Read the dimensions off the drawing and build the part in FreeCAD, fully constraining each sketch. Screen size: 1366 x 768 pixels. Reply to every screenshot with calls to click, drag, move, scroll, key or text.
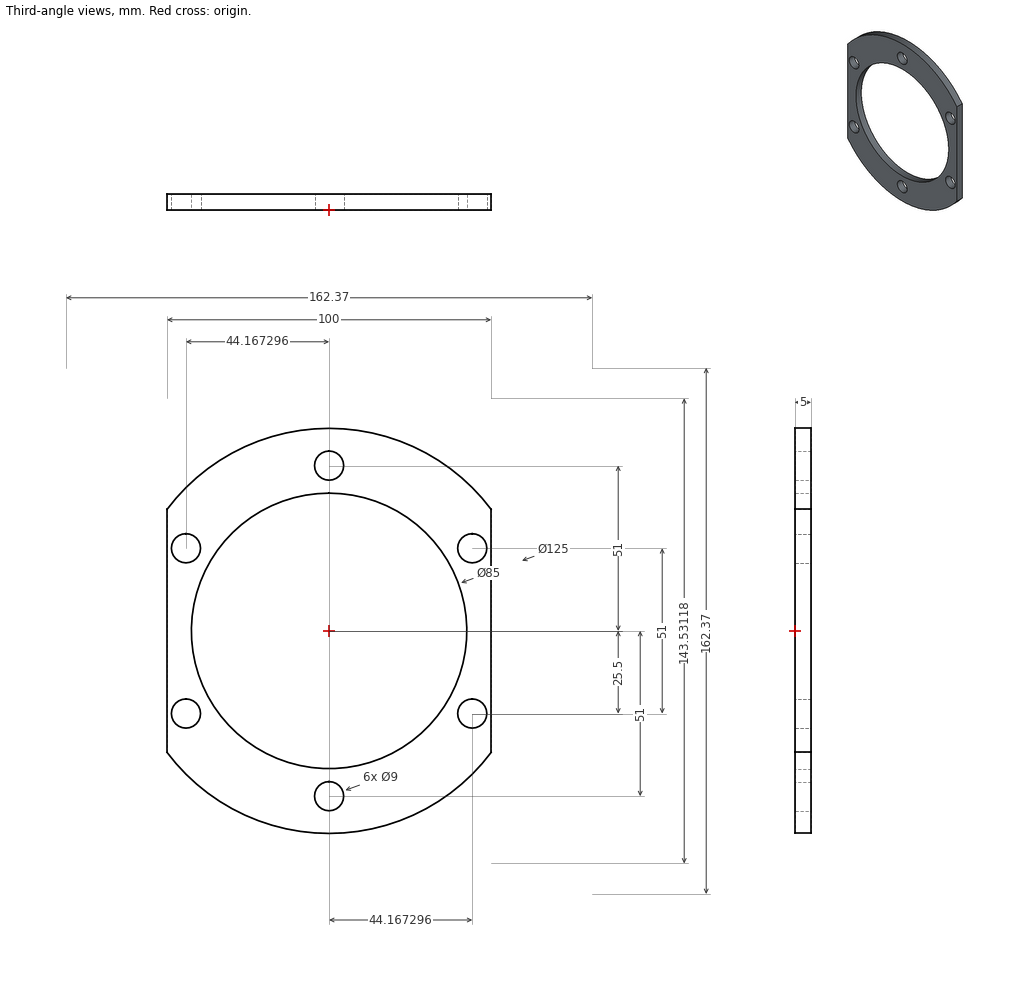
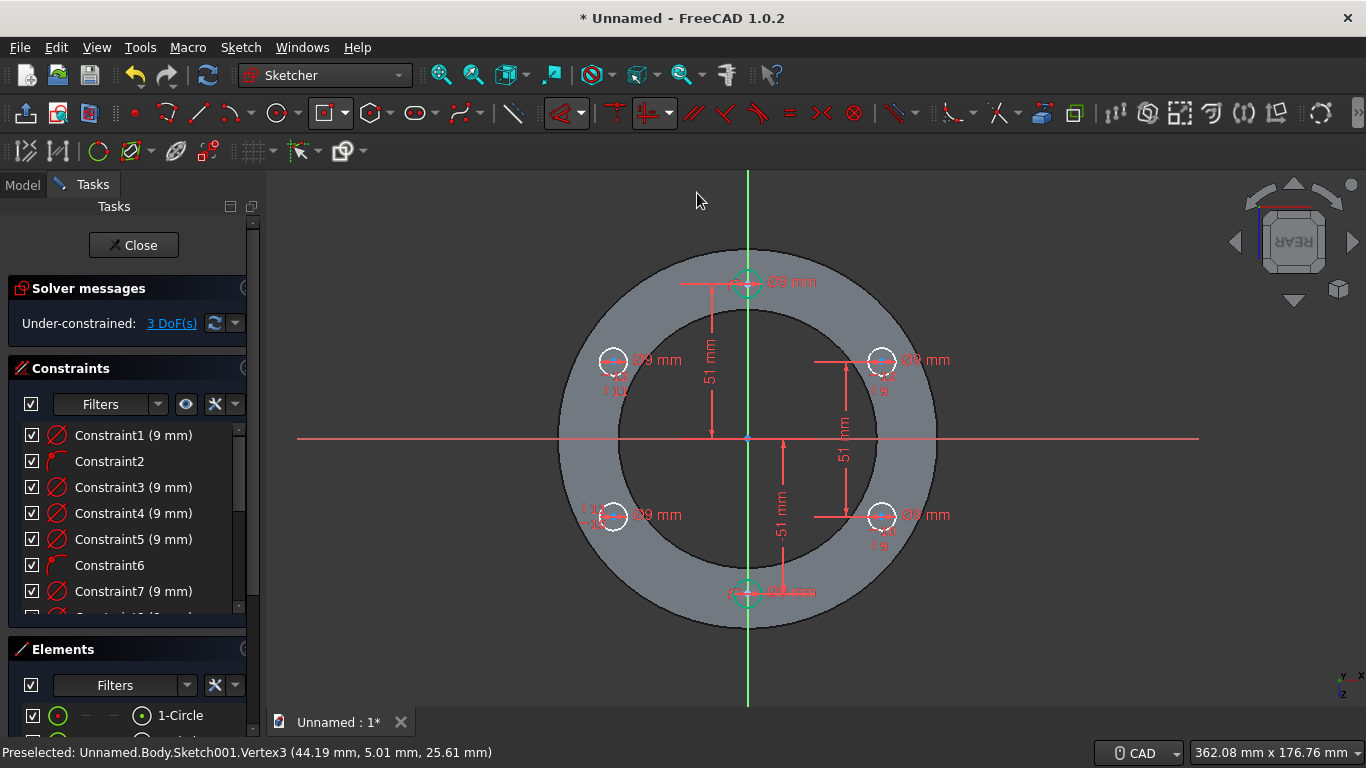
click(882, 362)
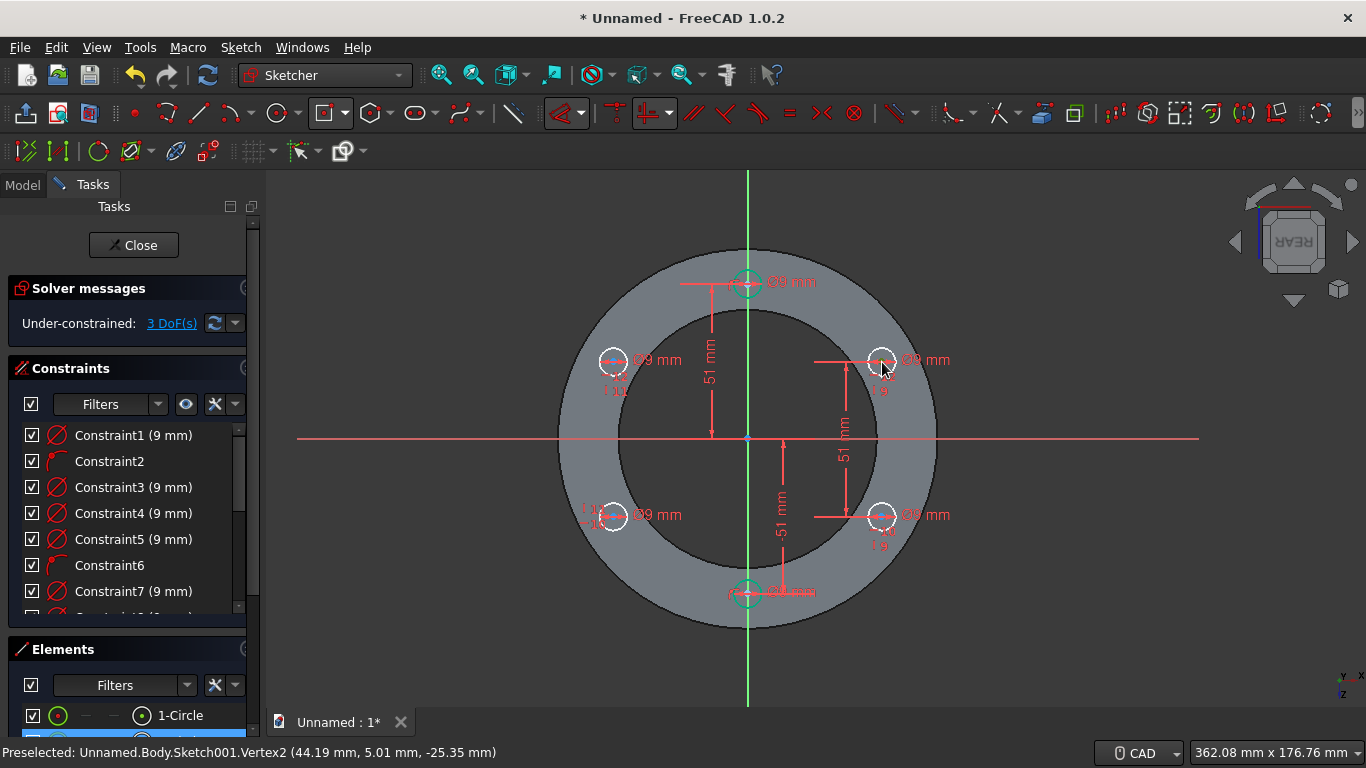
key(i)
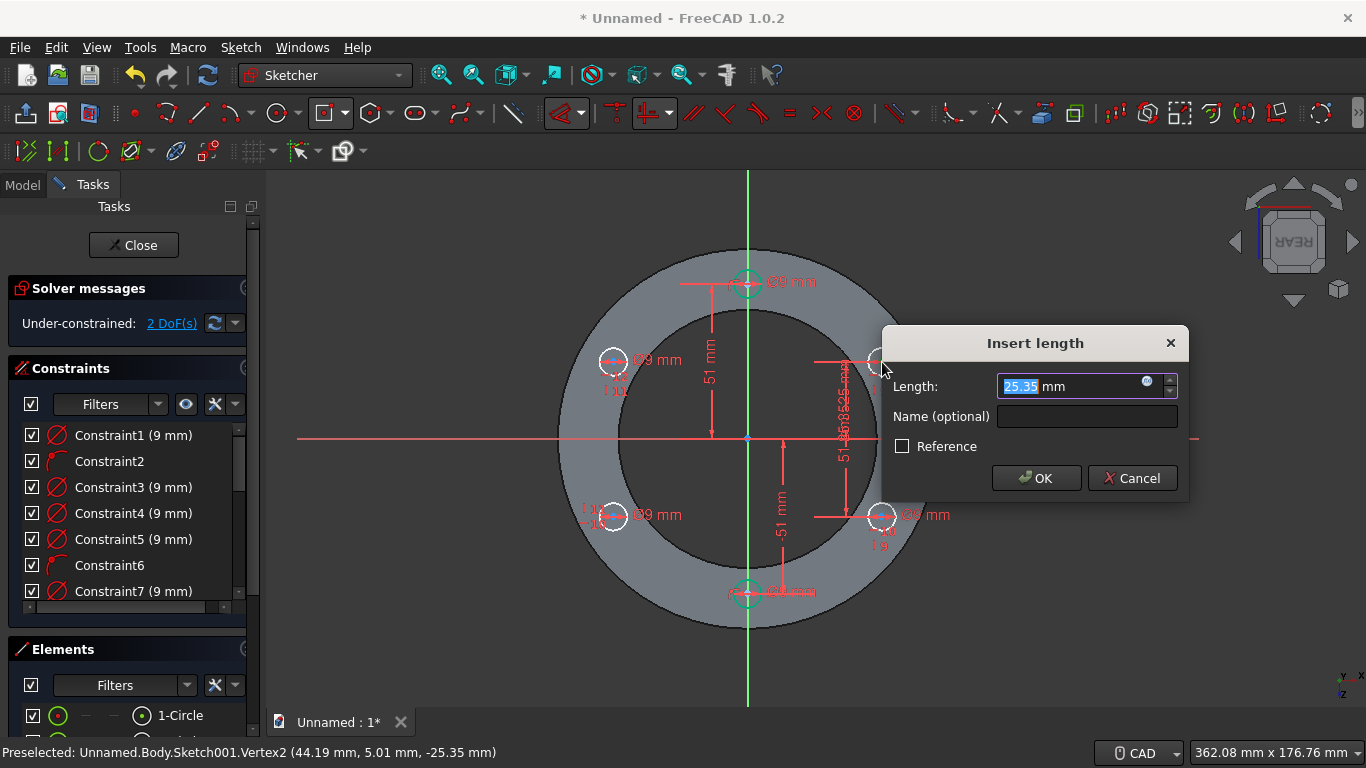
text(25.5)
key(Return)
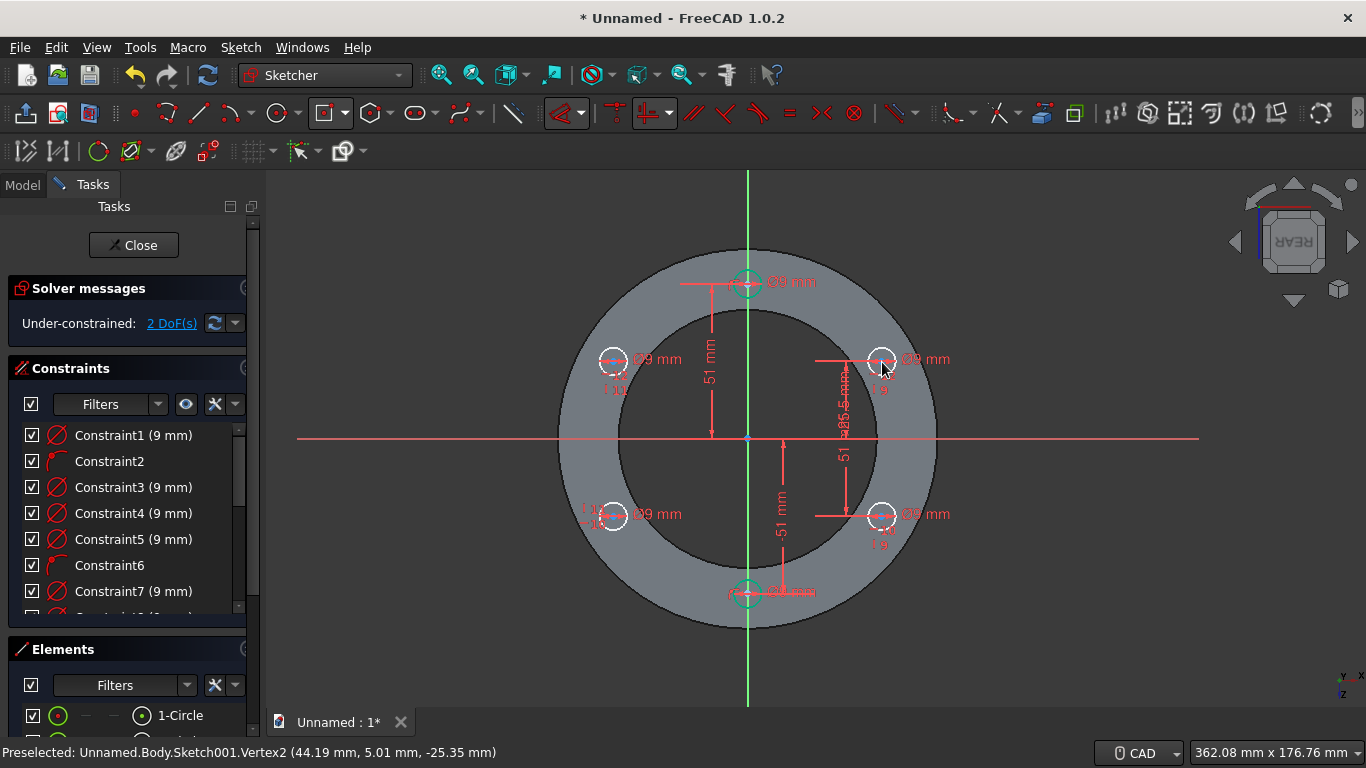
click(882, 361)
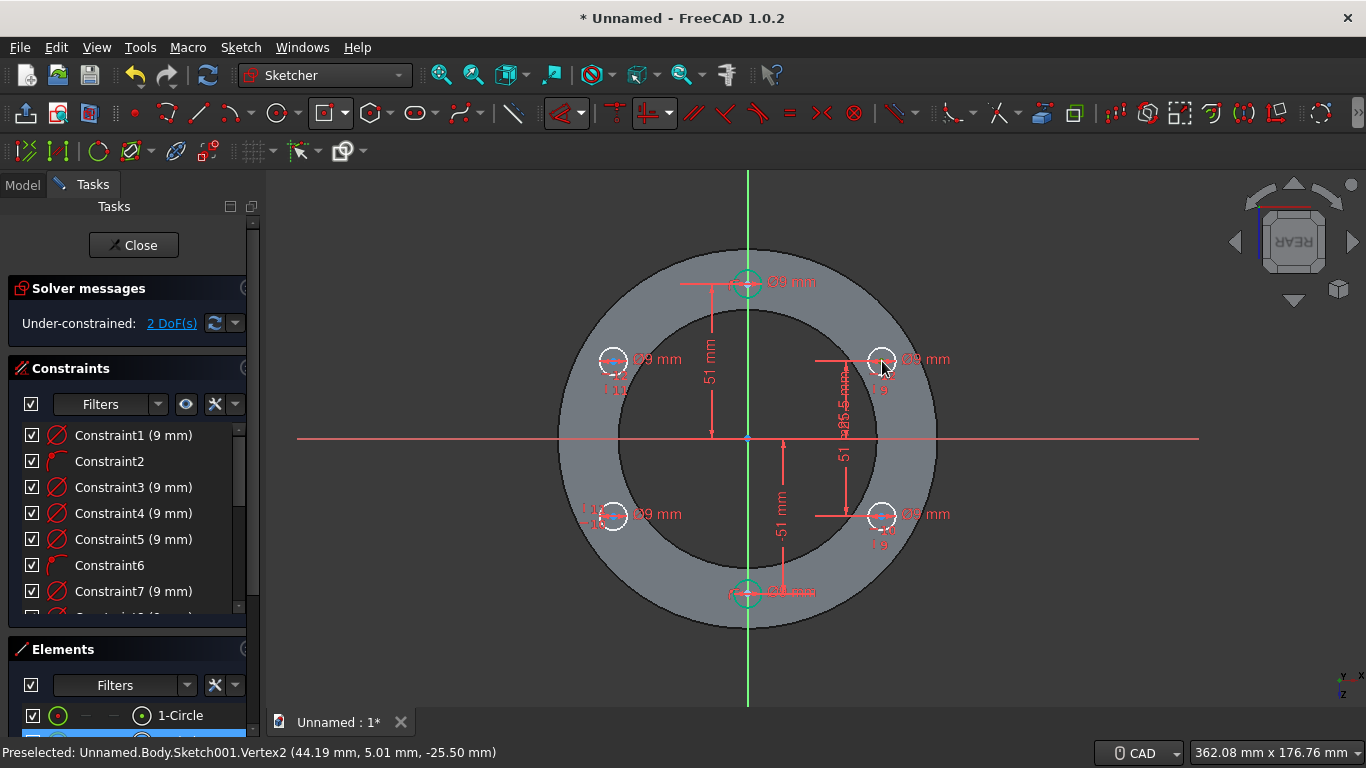
click(584, 114)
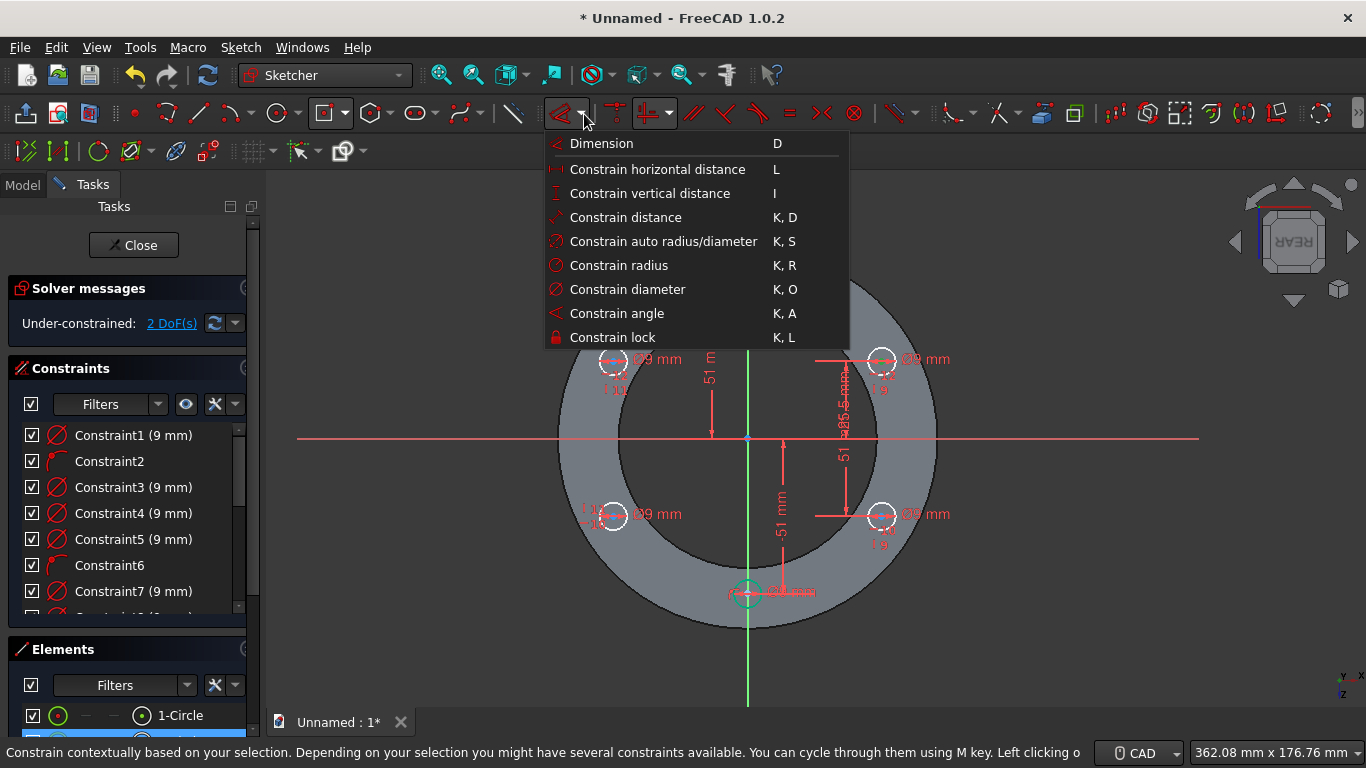
click(697, 169)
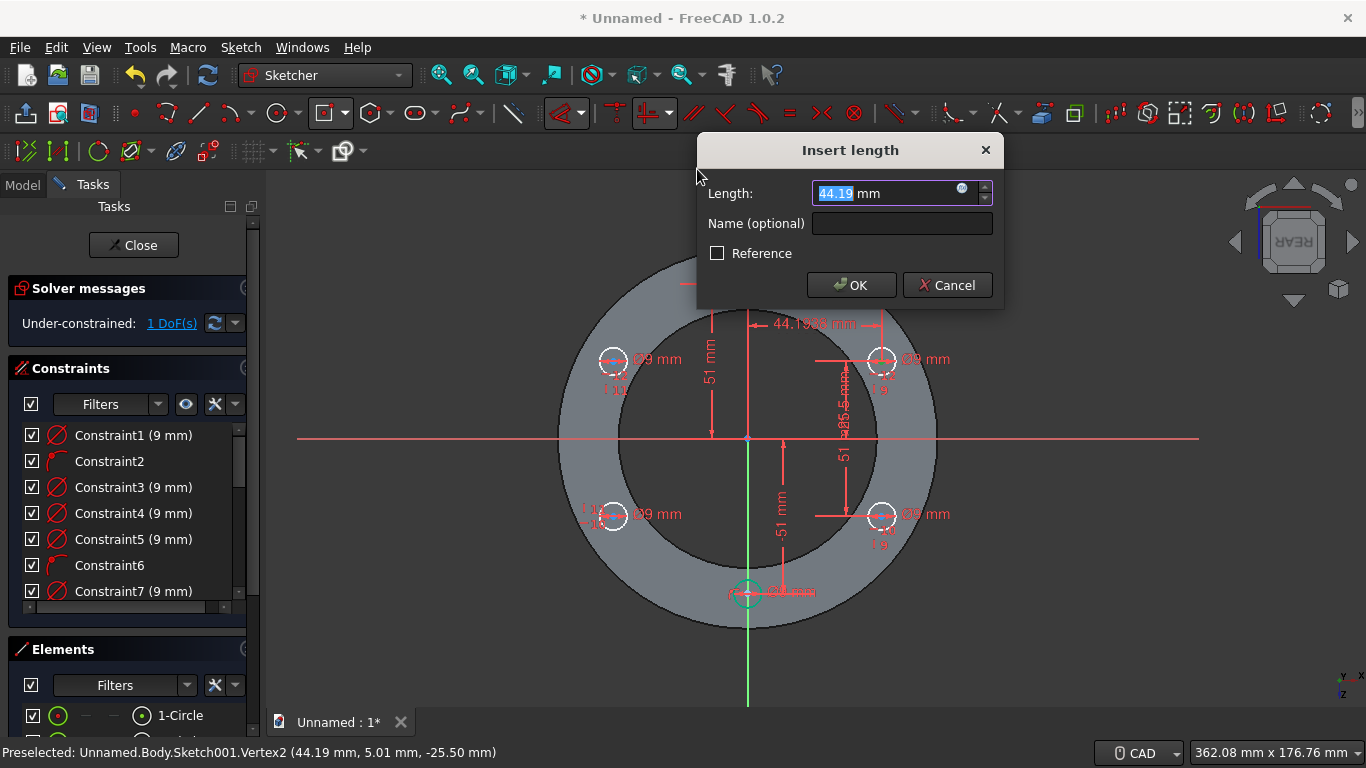
text(44.167296)
key(Return)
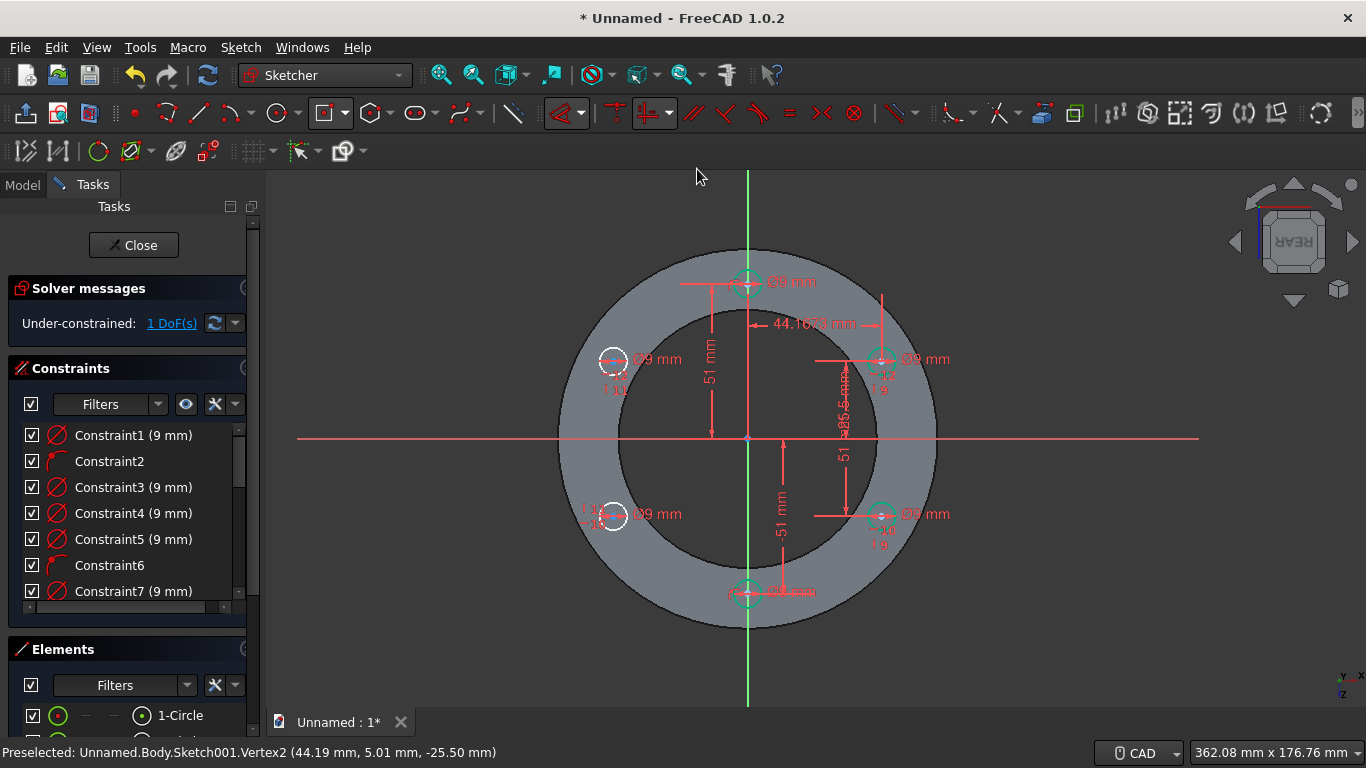
click(613, 516)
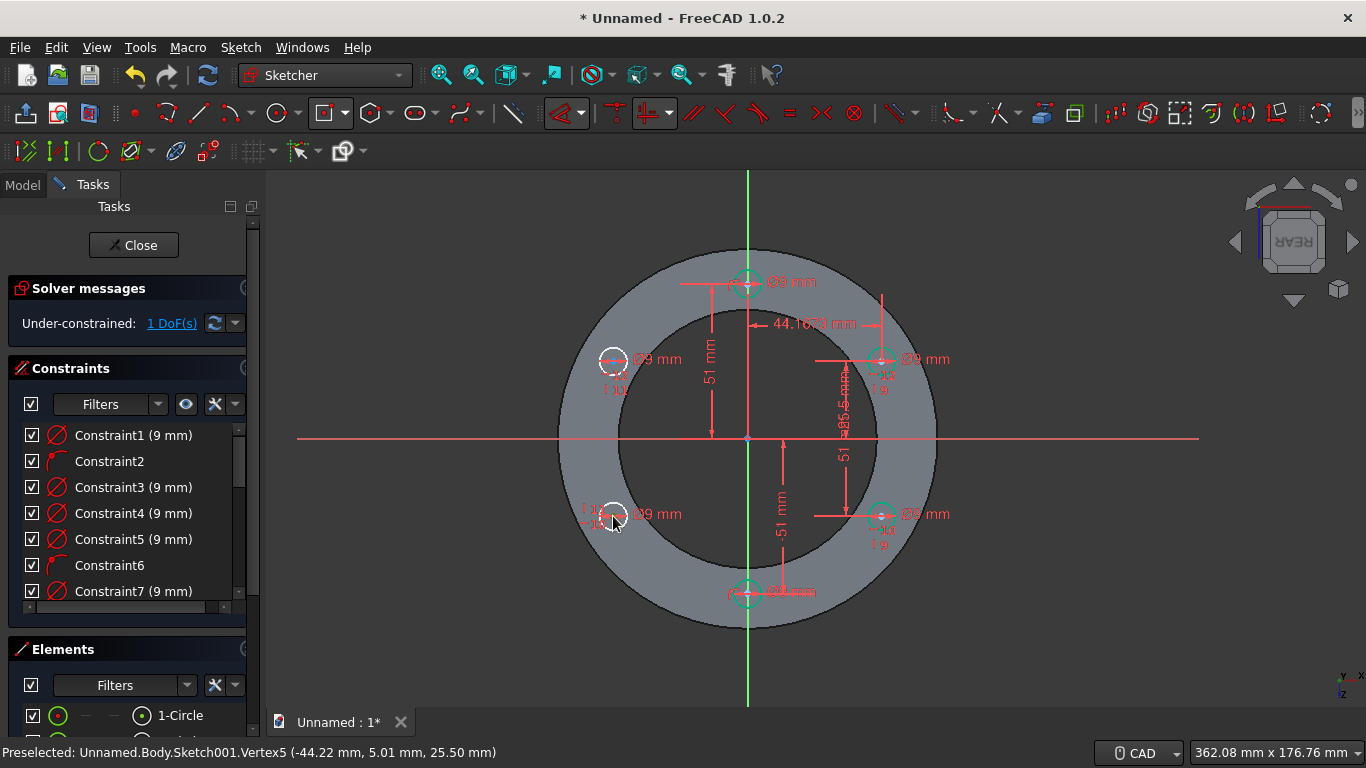
click(584, 114)